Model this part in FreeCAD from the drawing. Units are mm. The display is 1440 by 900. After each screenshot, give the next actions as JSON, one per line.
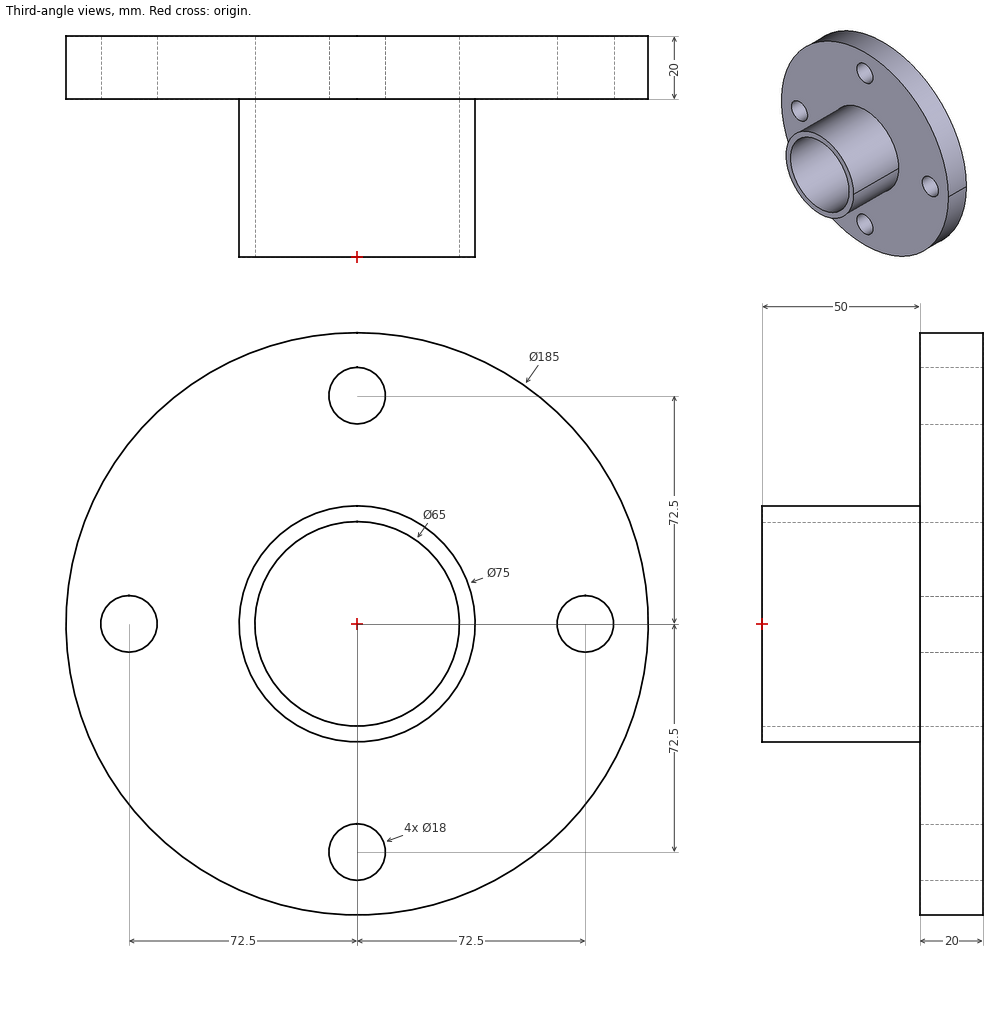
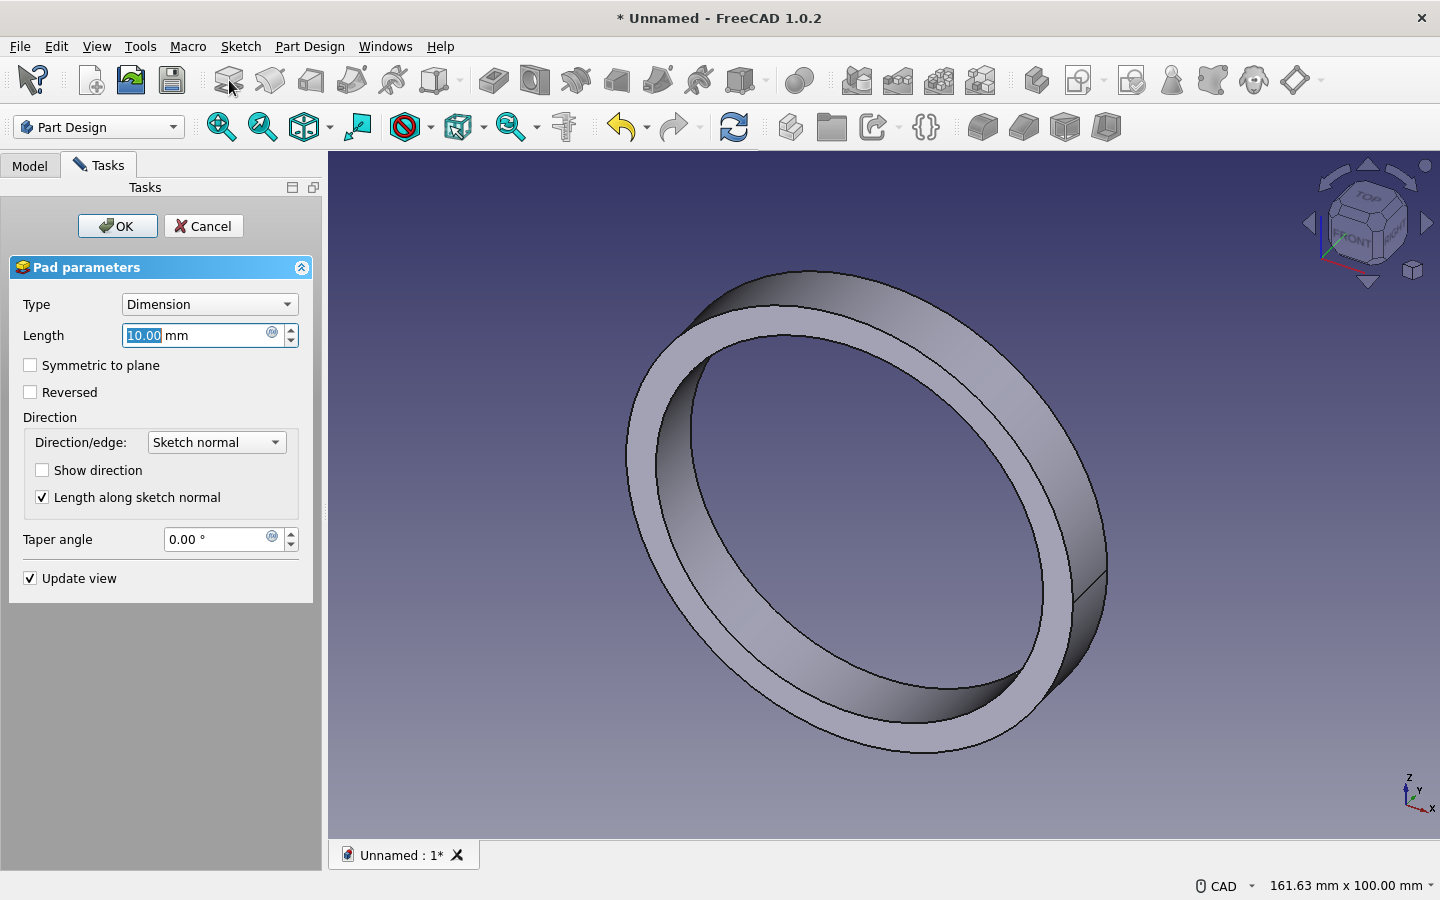
{"action": "type", "text": "50"}
{"action": "key", "text": "Tab"}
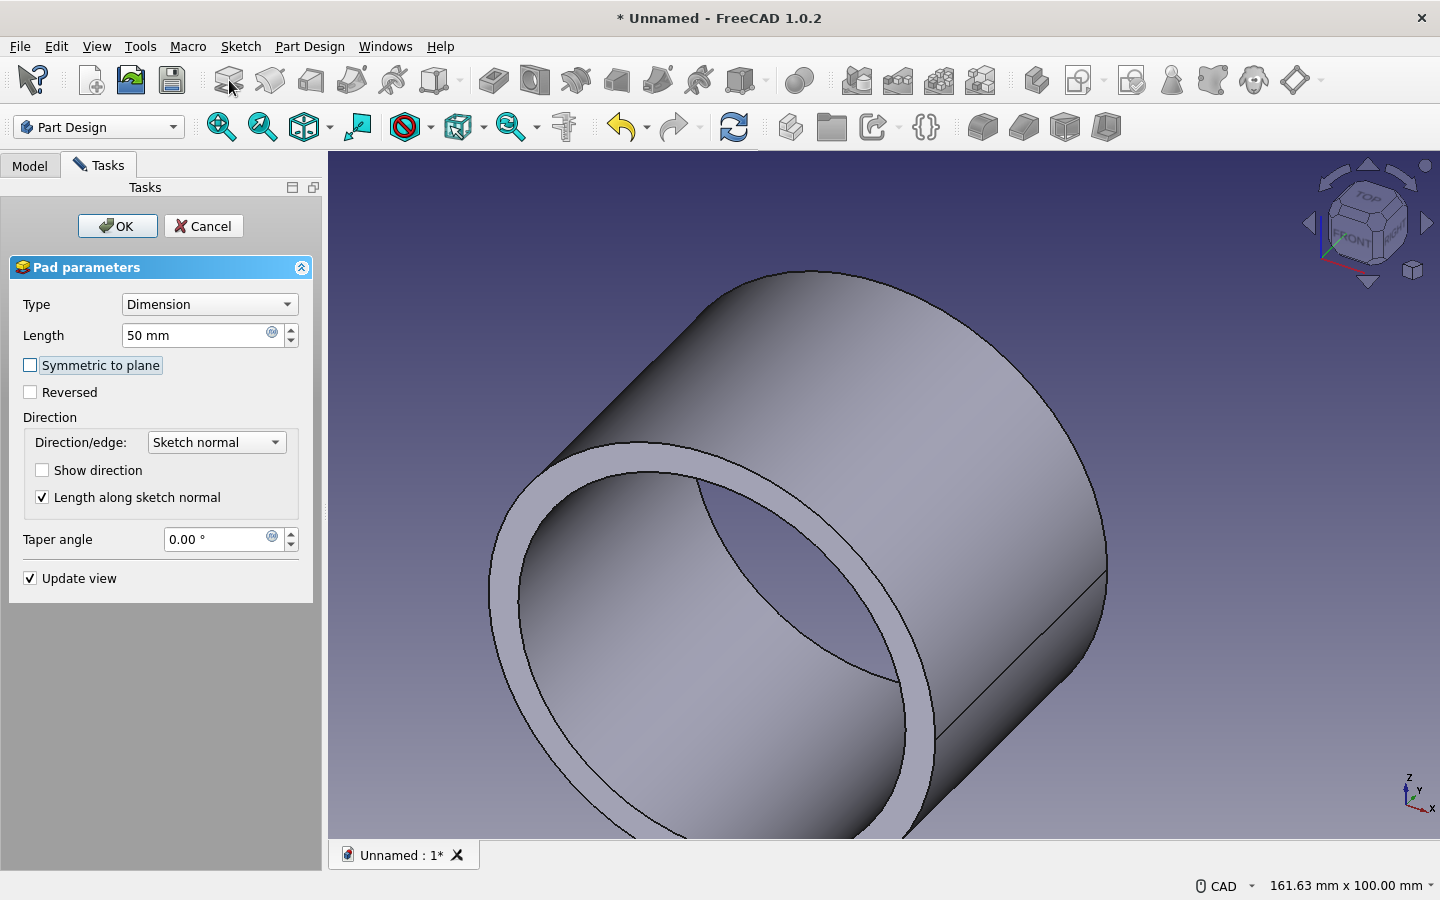
{"action": "left_click", "coordinate": [31, 392]}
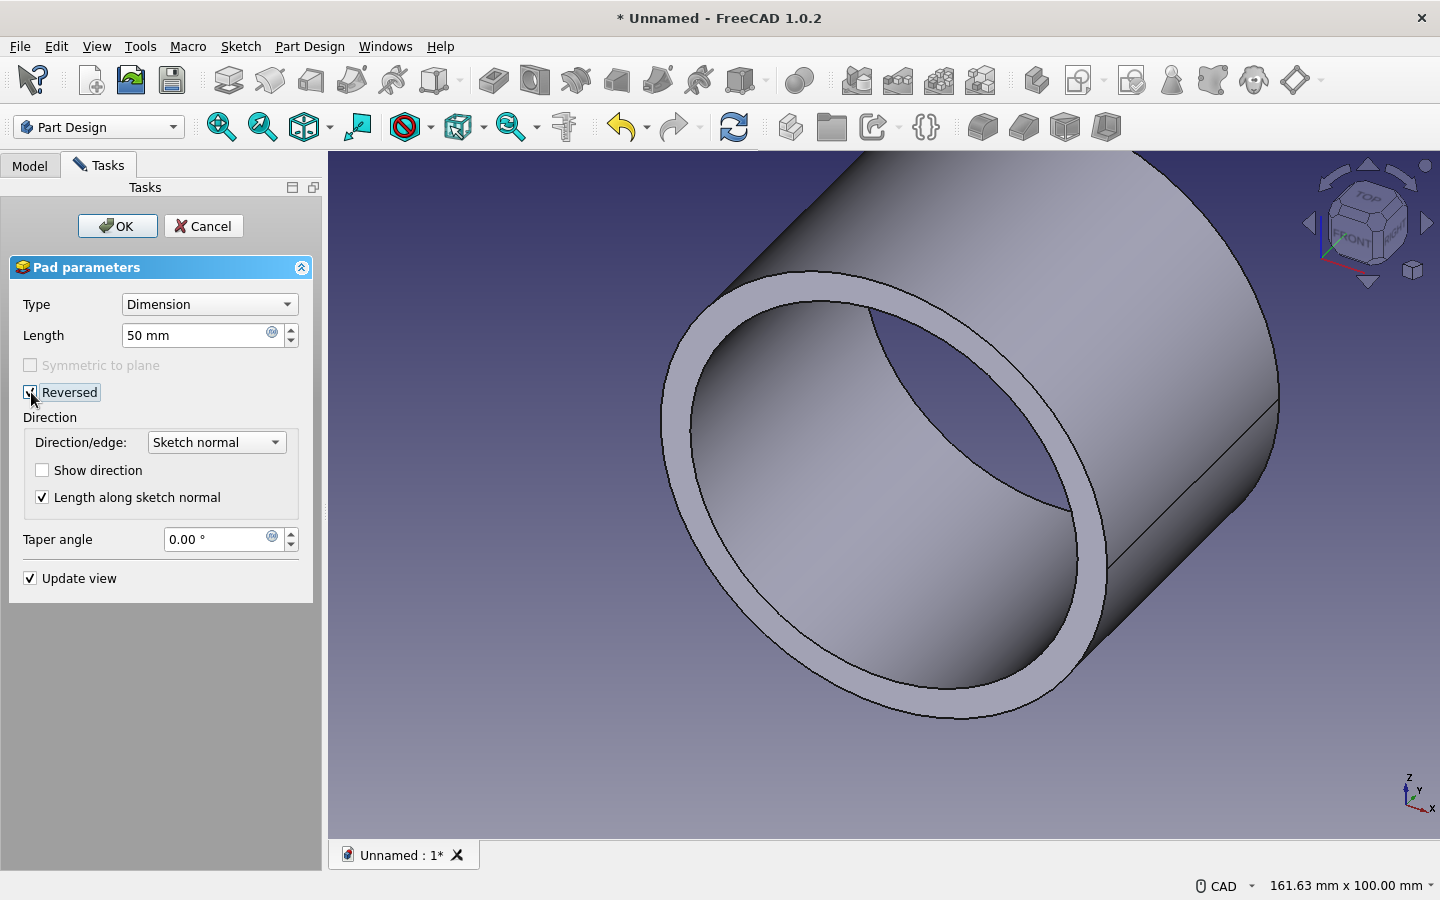
{"action": "left_click", "coordinate": [118, 226]}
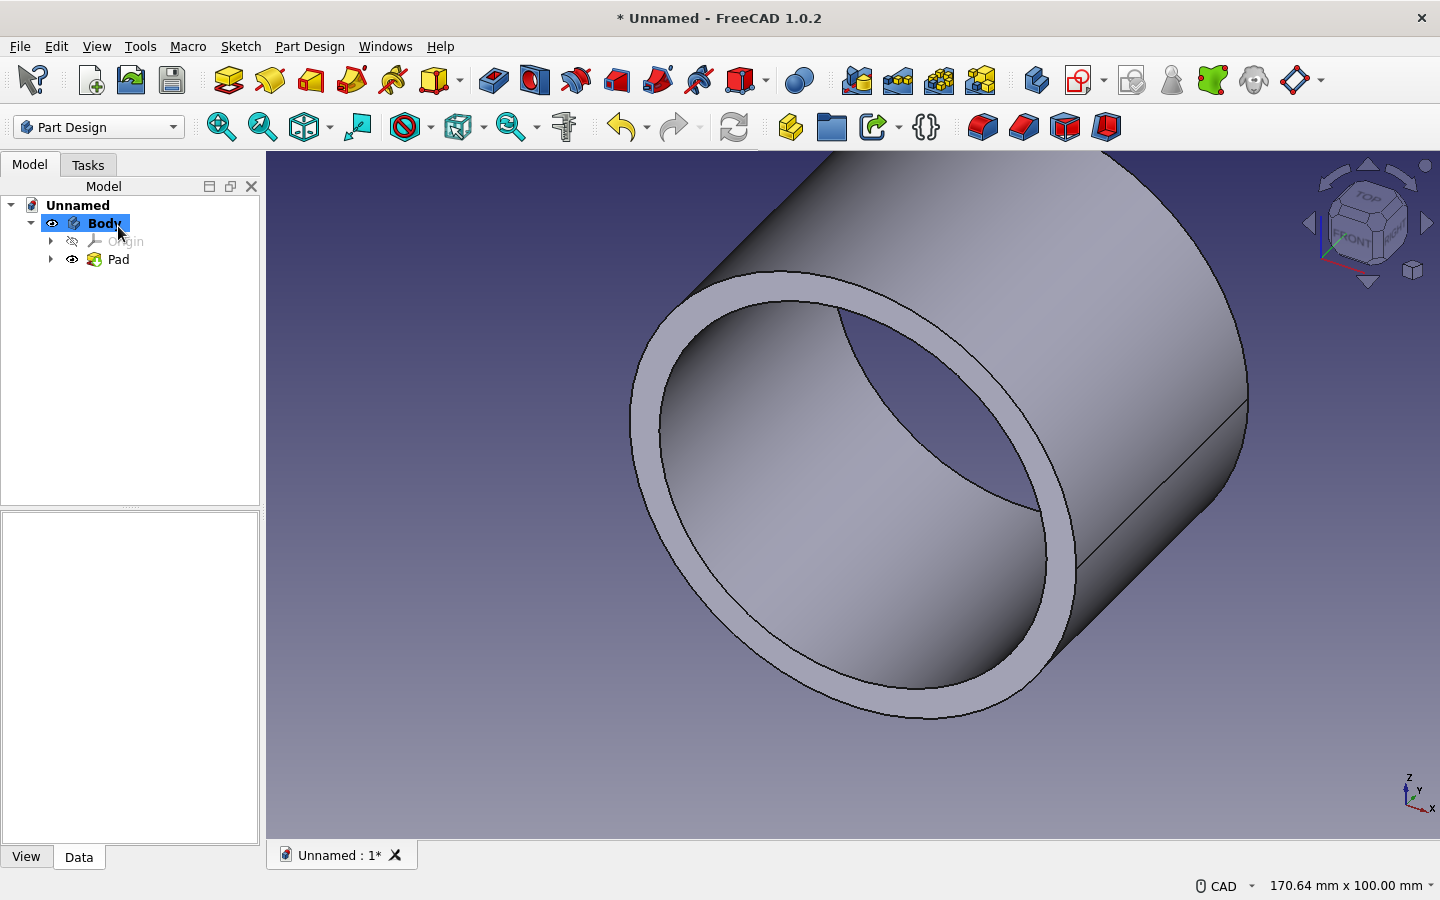
{"action": "left_click", "coordinate": [222, 128]}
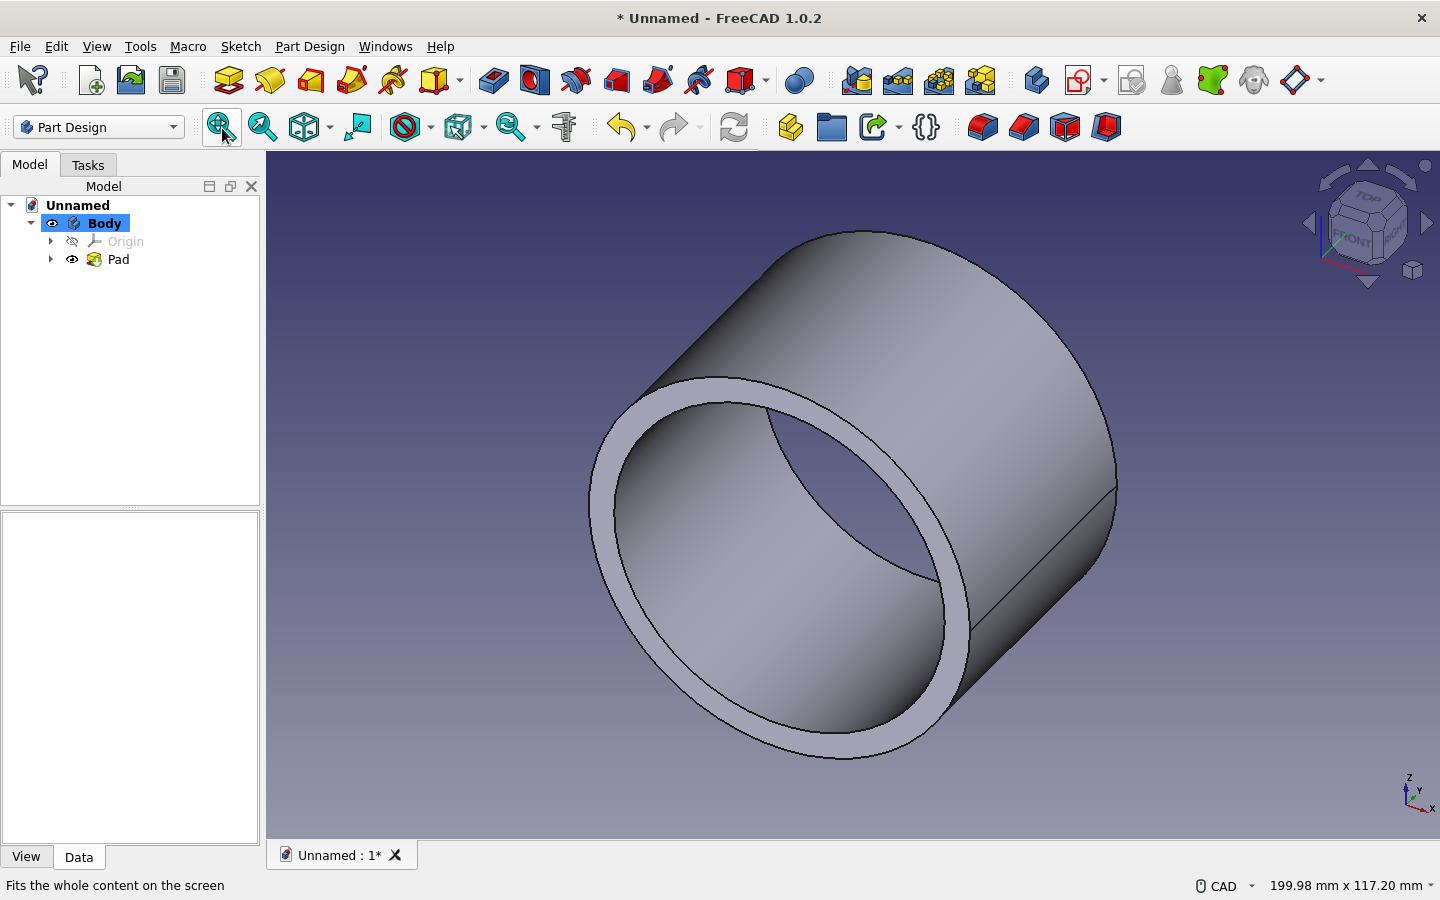
{"action": "left_click", "coordinate": [1037, 80]}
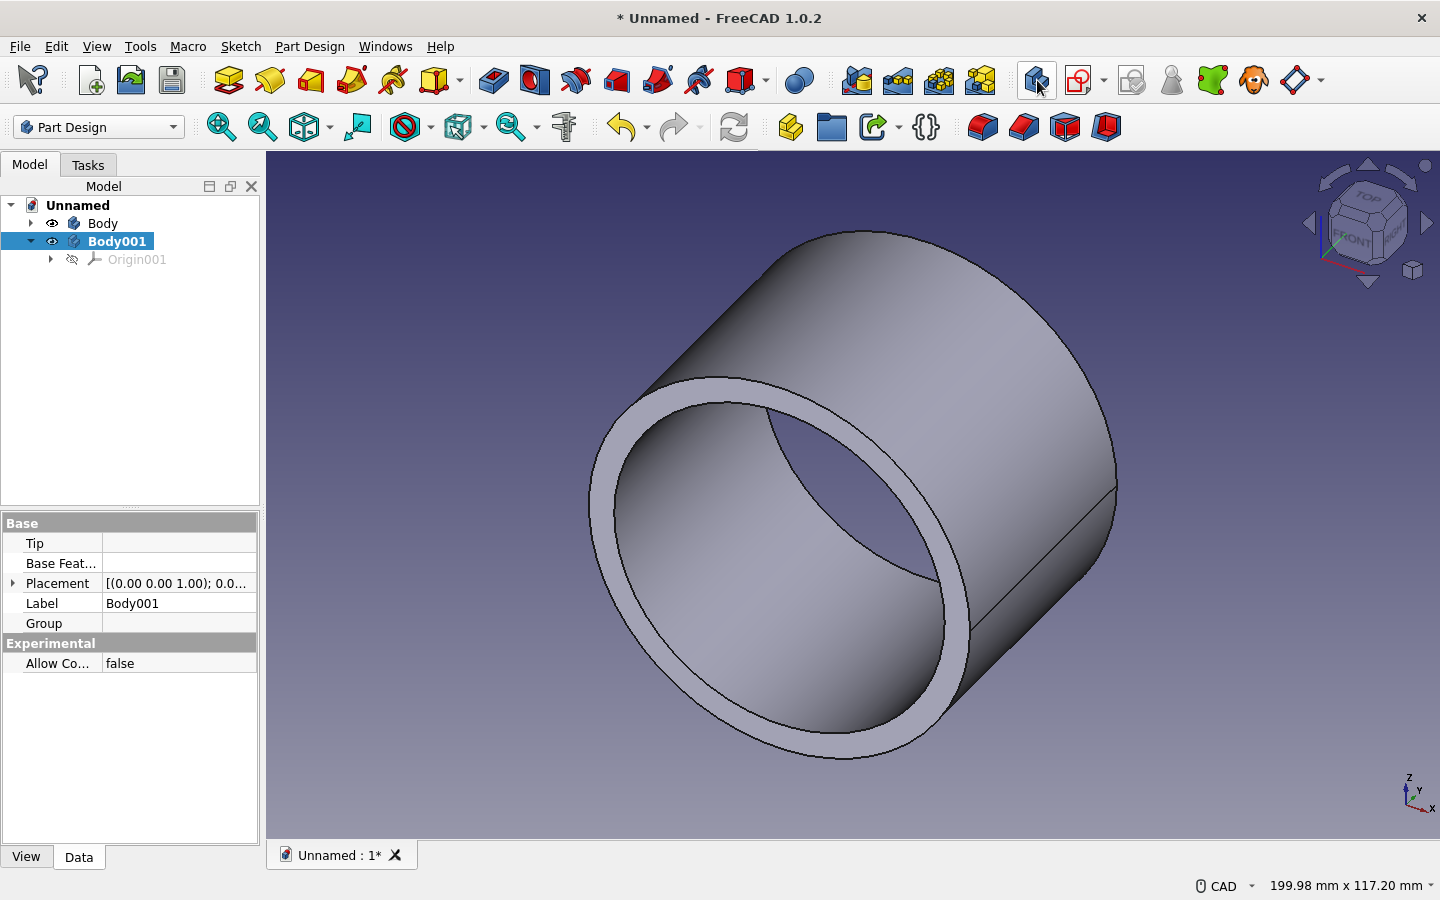
{"action": "left_click", "coordinate": [51, 259]}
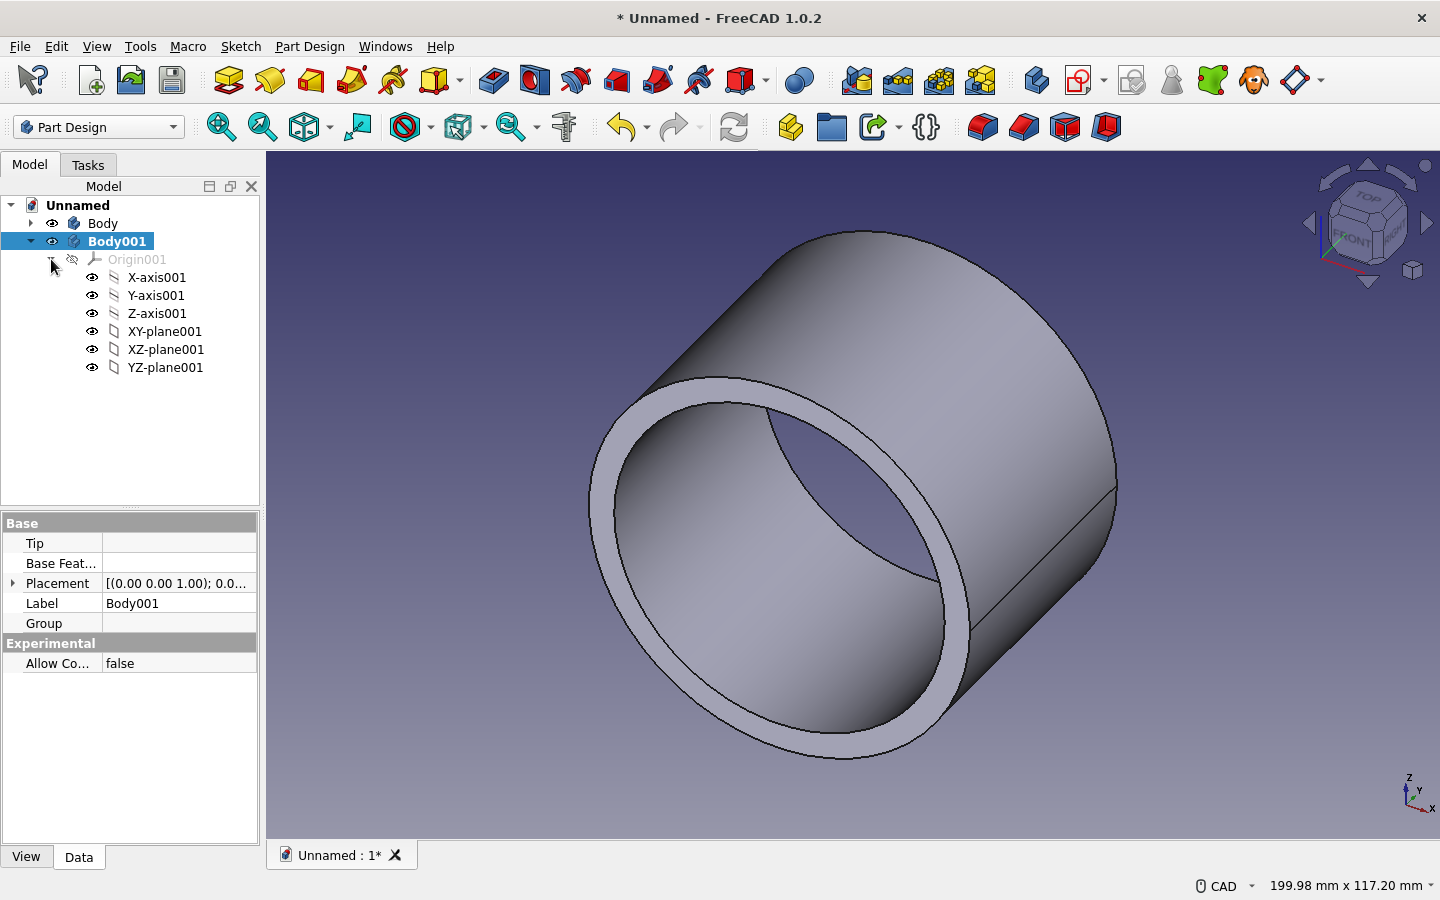
{"action": "left_click", "coordinate": [137, 349]}